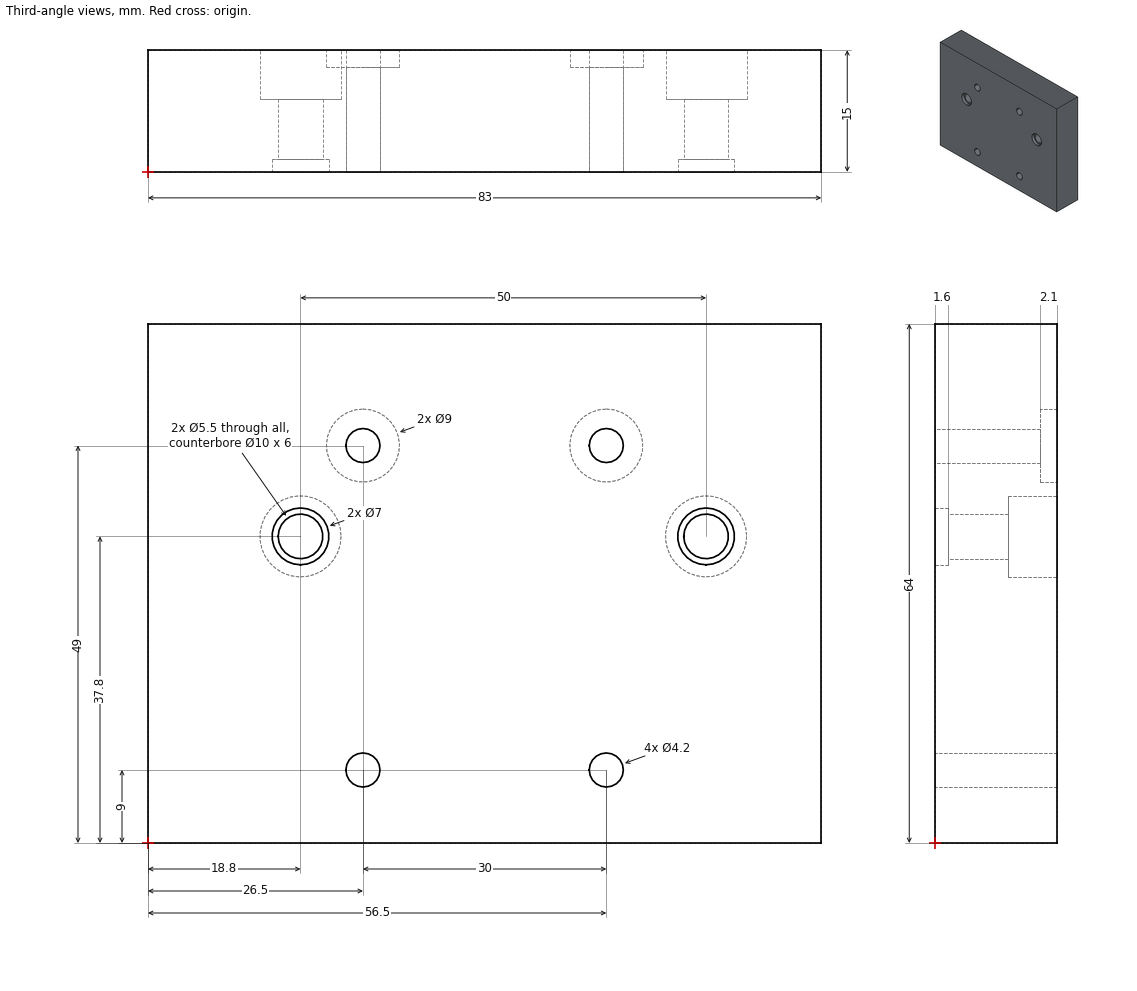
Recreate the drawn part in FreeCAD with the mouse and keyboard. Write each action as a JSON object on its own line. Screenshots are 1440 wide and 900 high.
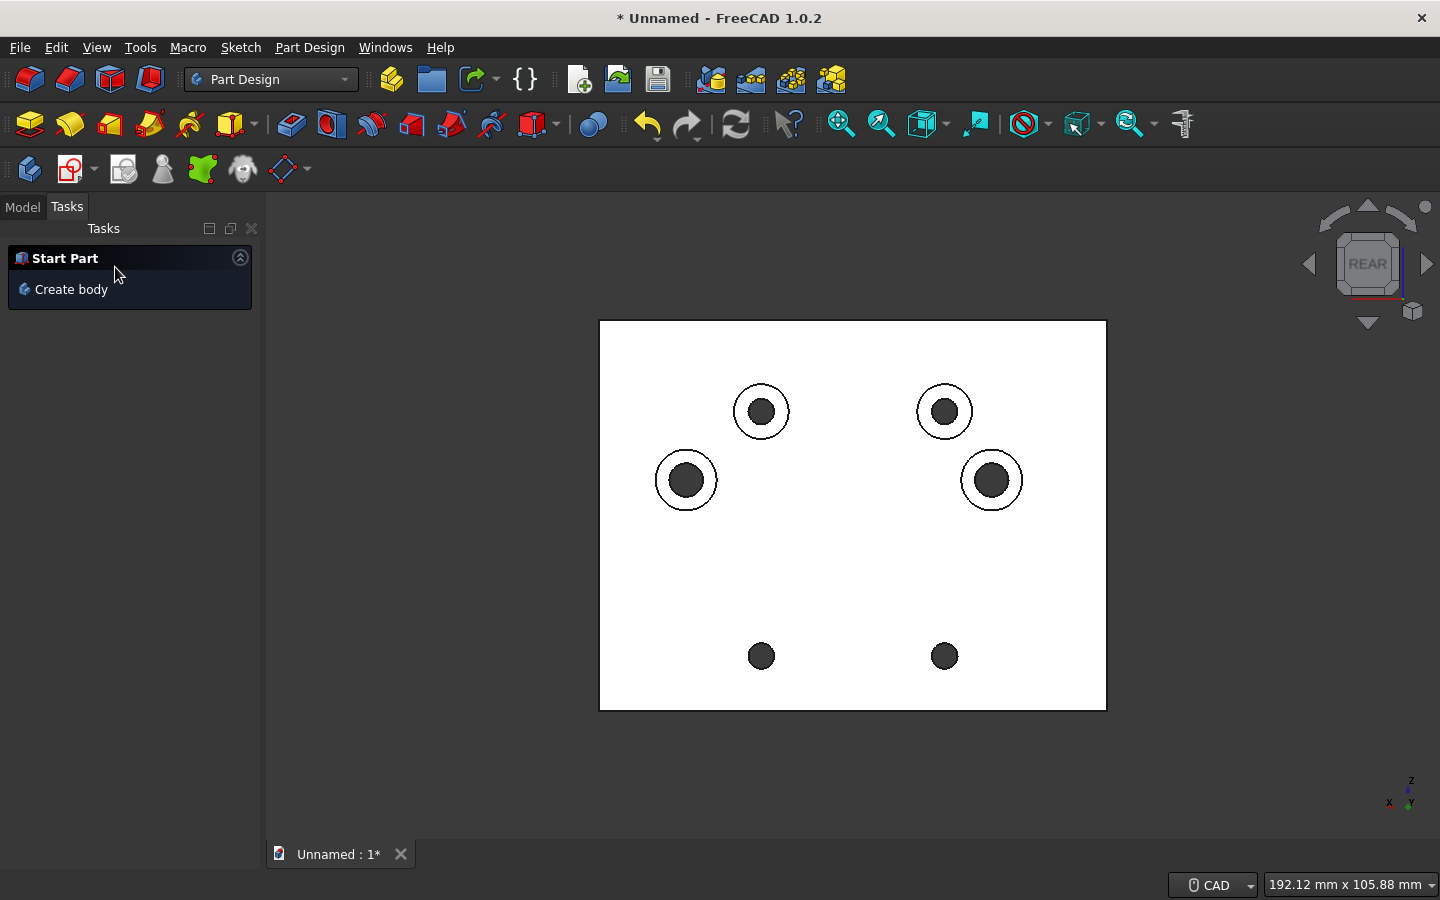
{"action": "key", "text": "0"}